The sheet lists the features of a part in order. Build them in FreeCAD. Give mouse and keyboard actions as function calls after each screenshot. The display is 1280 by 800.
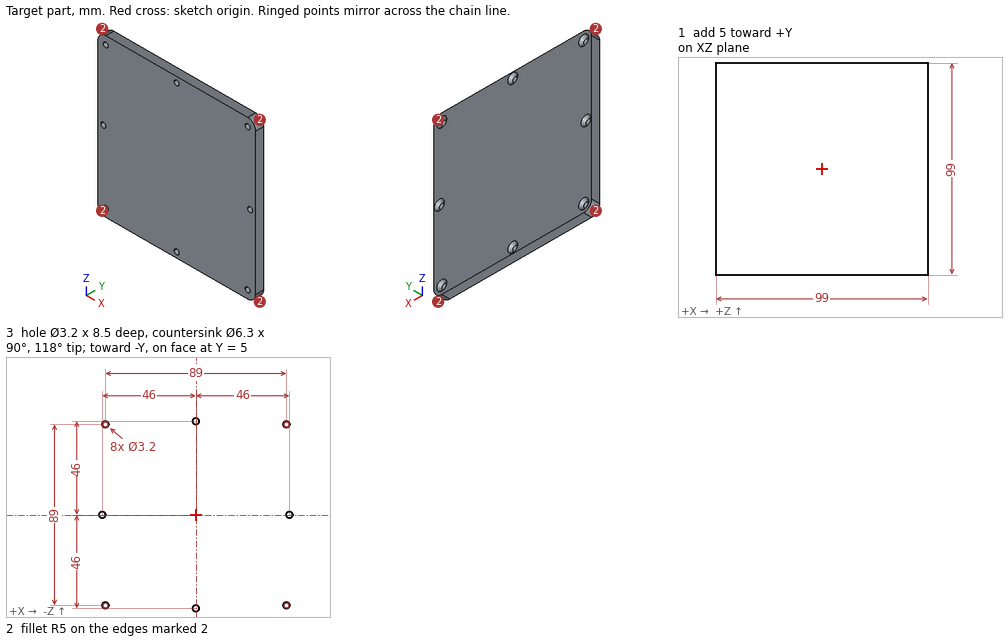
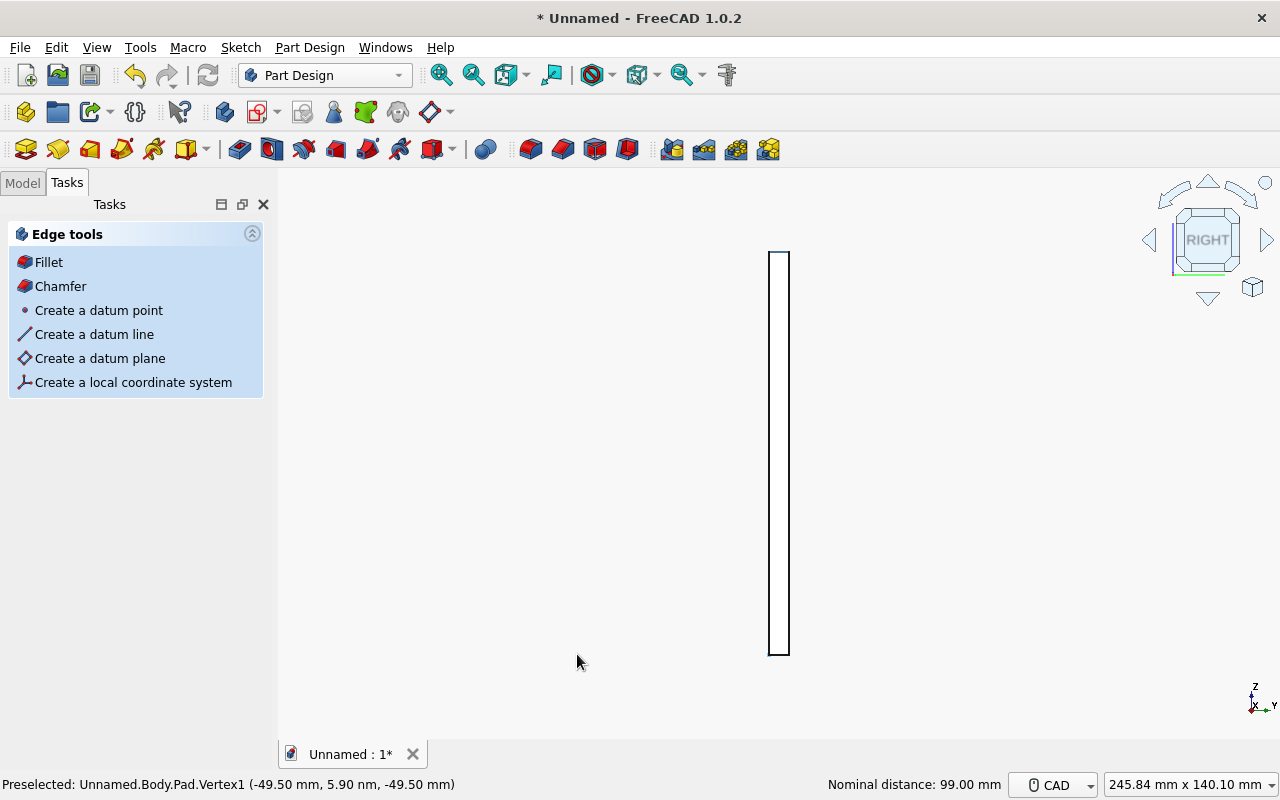
click(779, 654, ctrl)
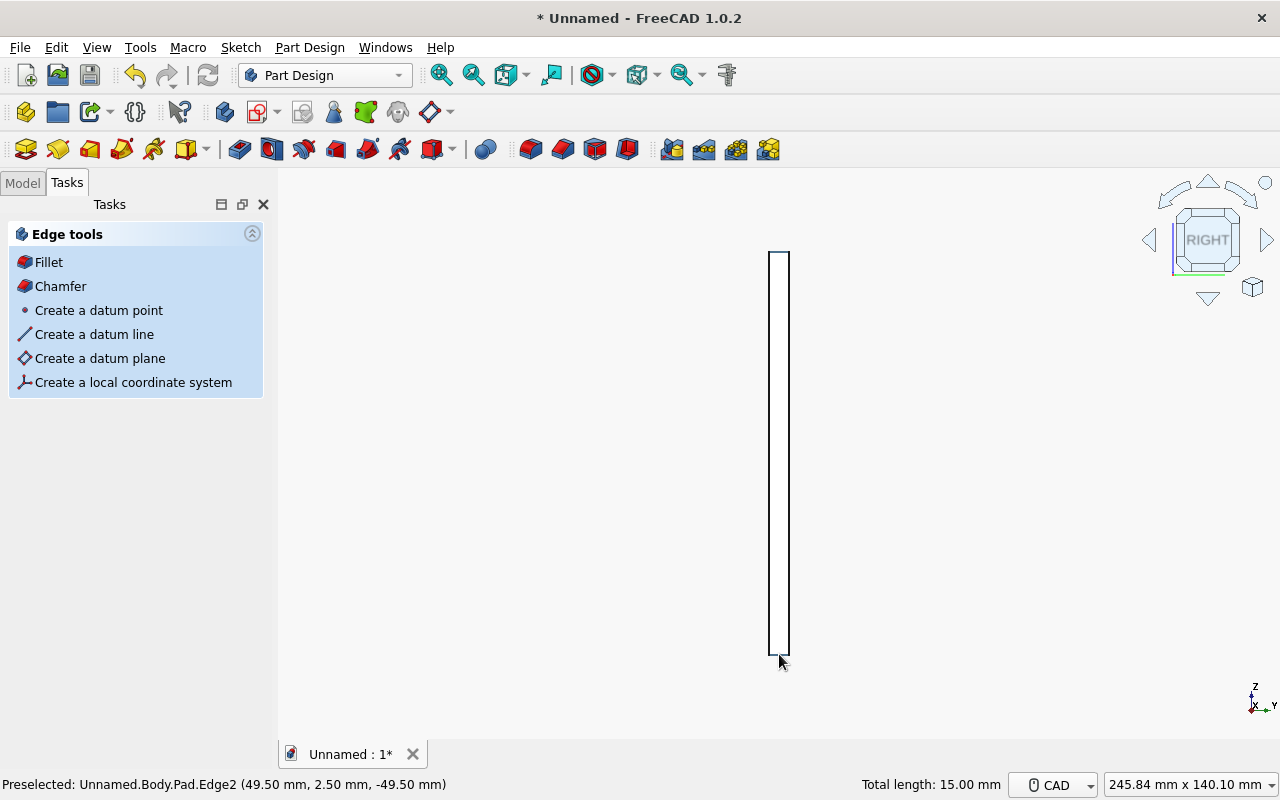
scroll(779, 654, up, 4)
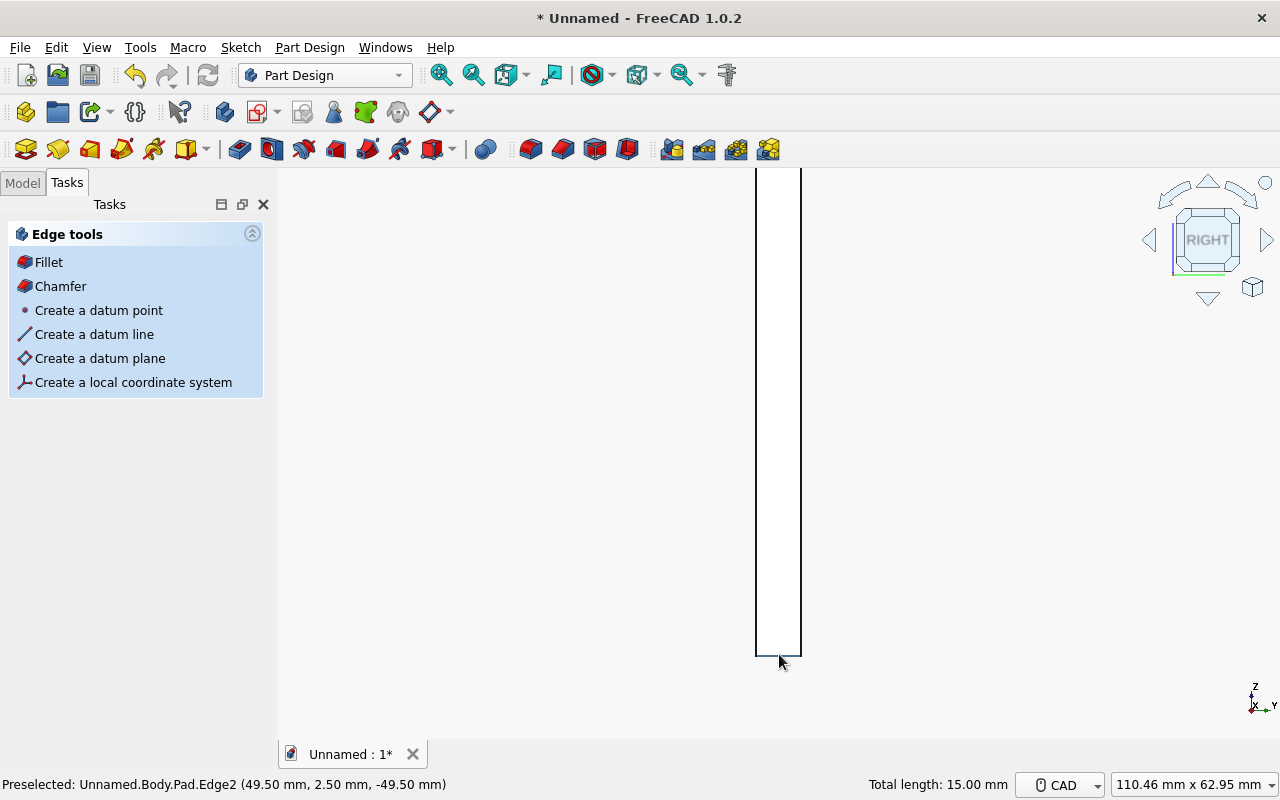
key(v)
key(f)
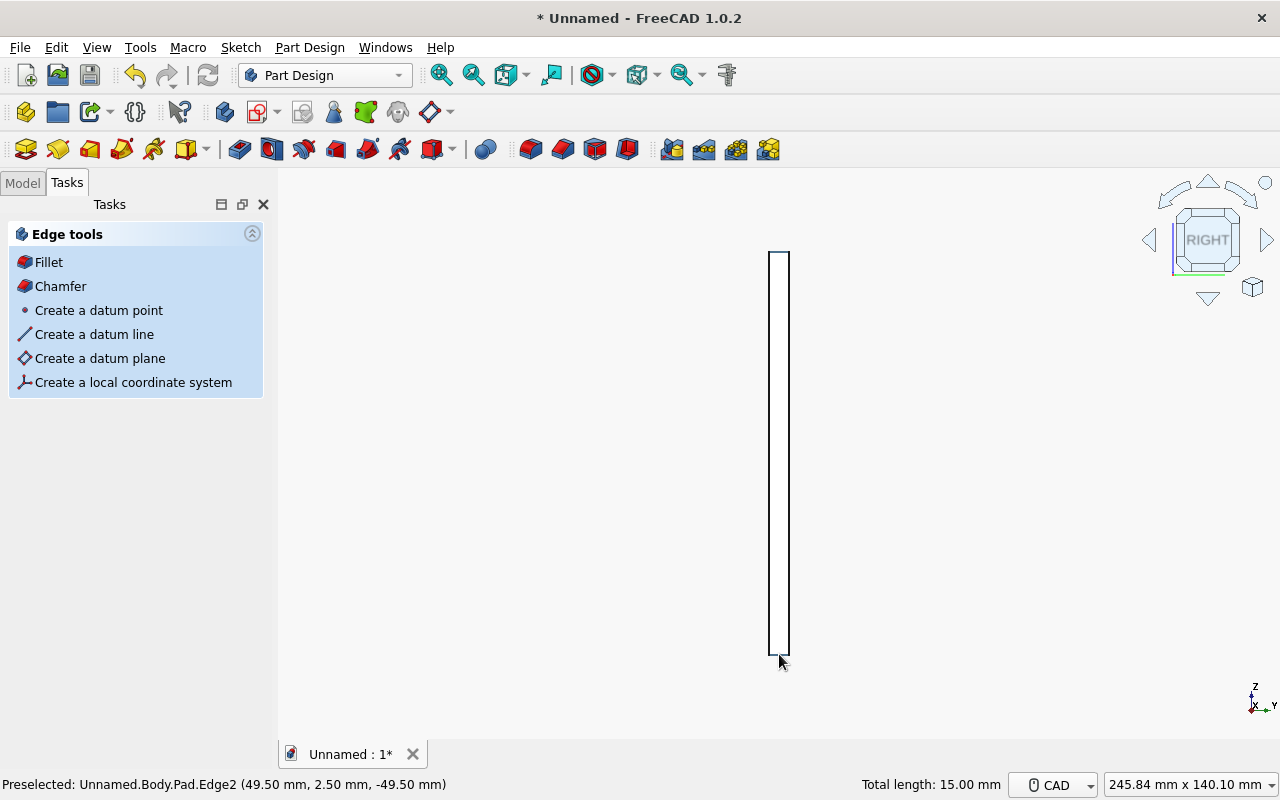
key(5)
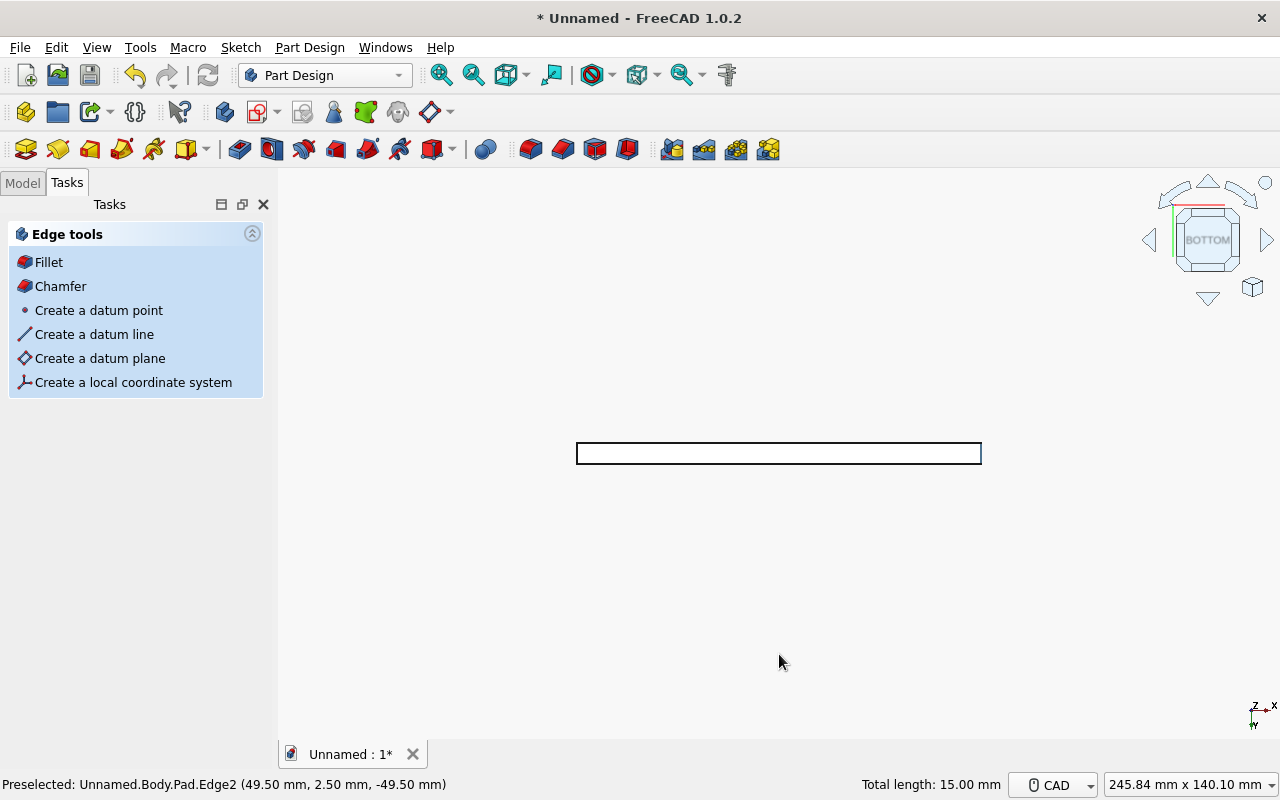
key(v)
key(f)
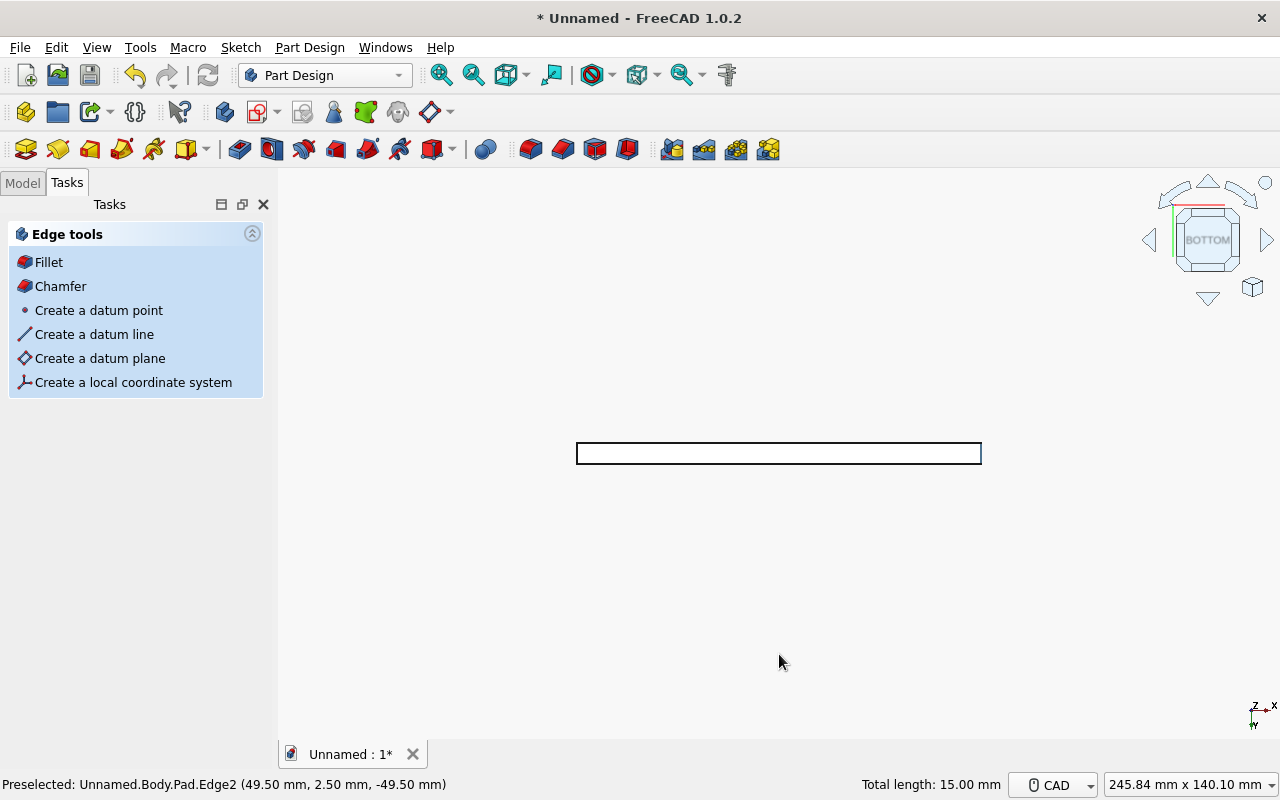
click(577, 452, ctrl)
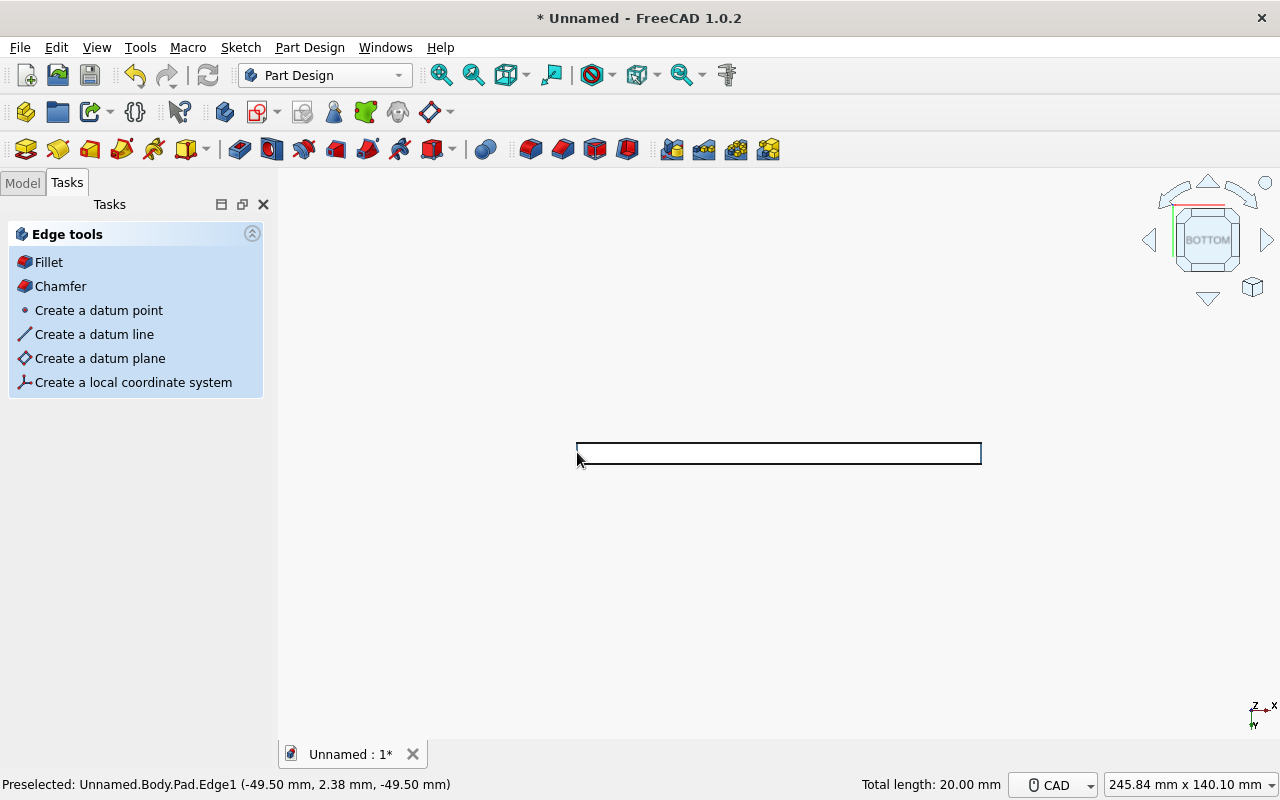
click(532, 150)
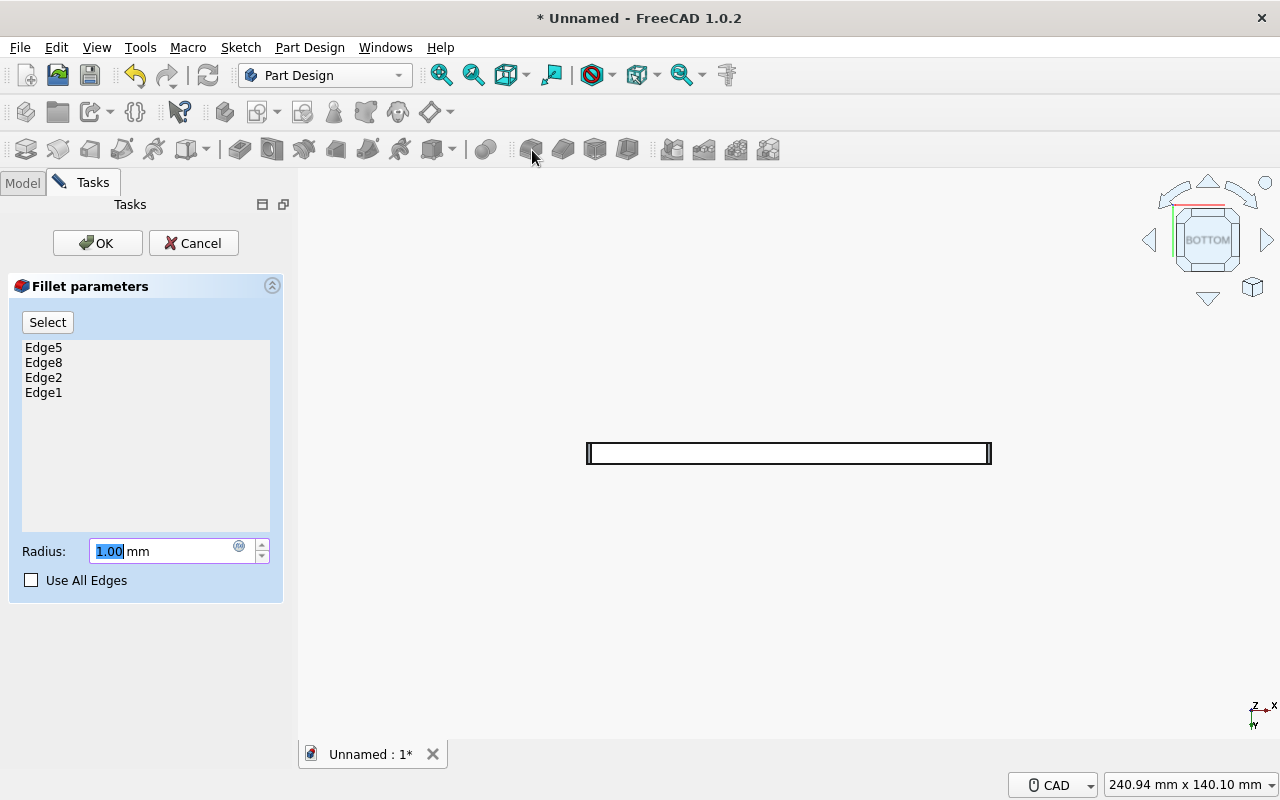
text(5)
key(Tab)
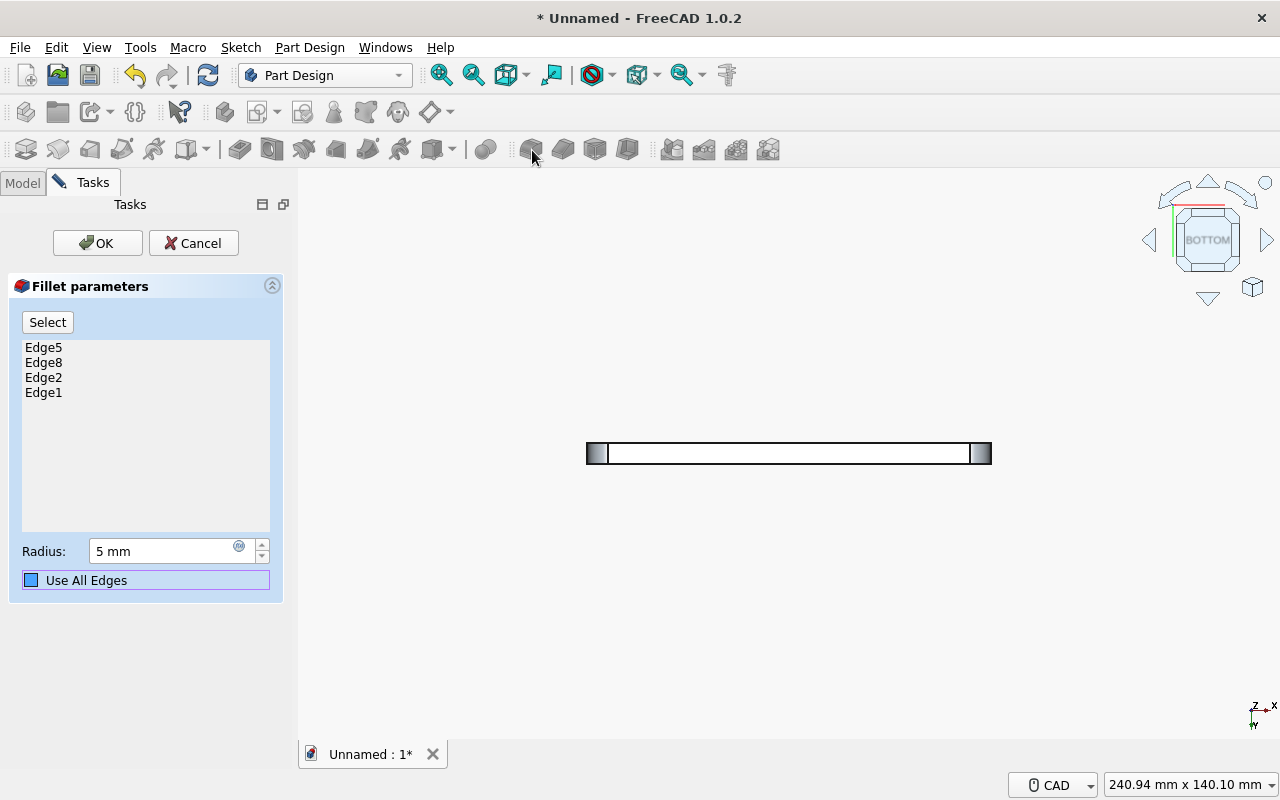
click(98, 243)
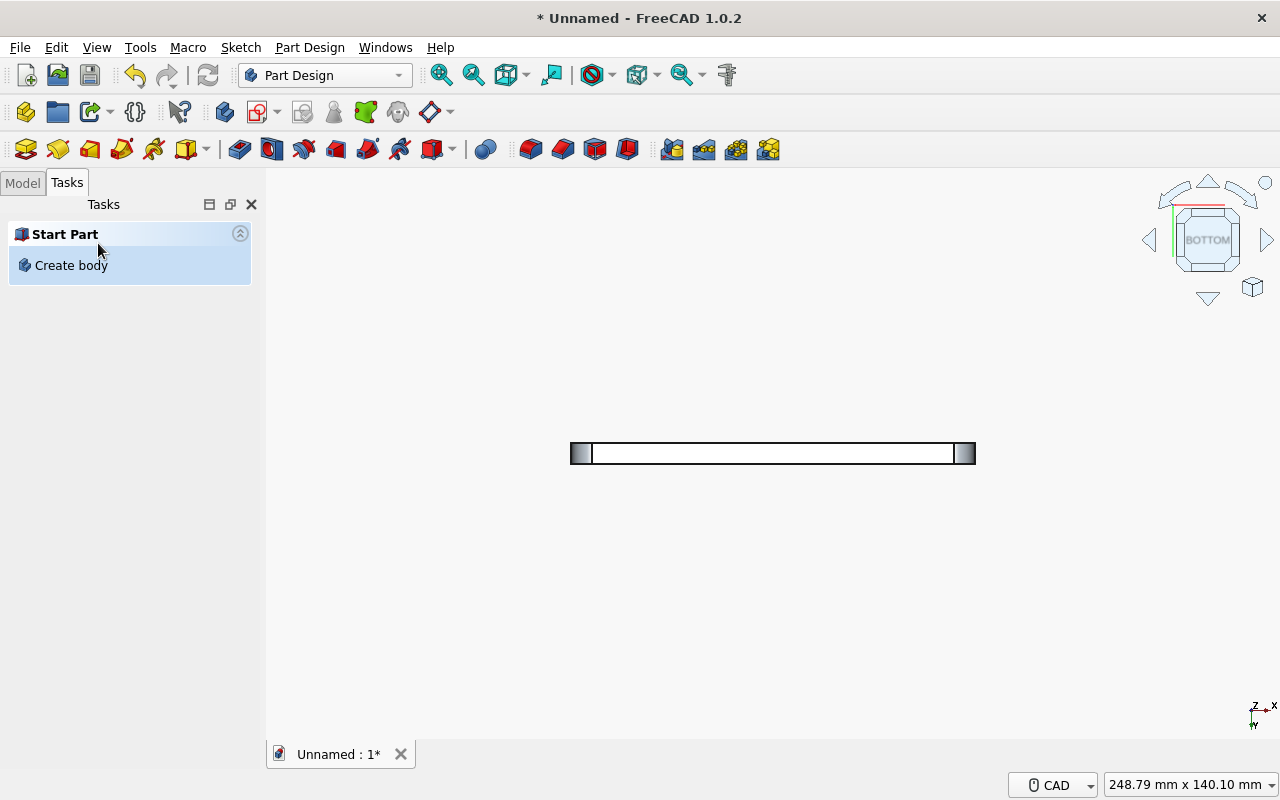
key(v)
key(f)